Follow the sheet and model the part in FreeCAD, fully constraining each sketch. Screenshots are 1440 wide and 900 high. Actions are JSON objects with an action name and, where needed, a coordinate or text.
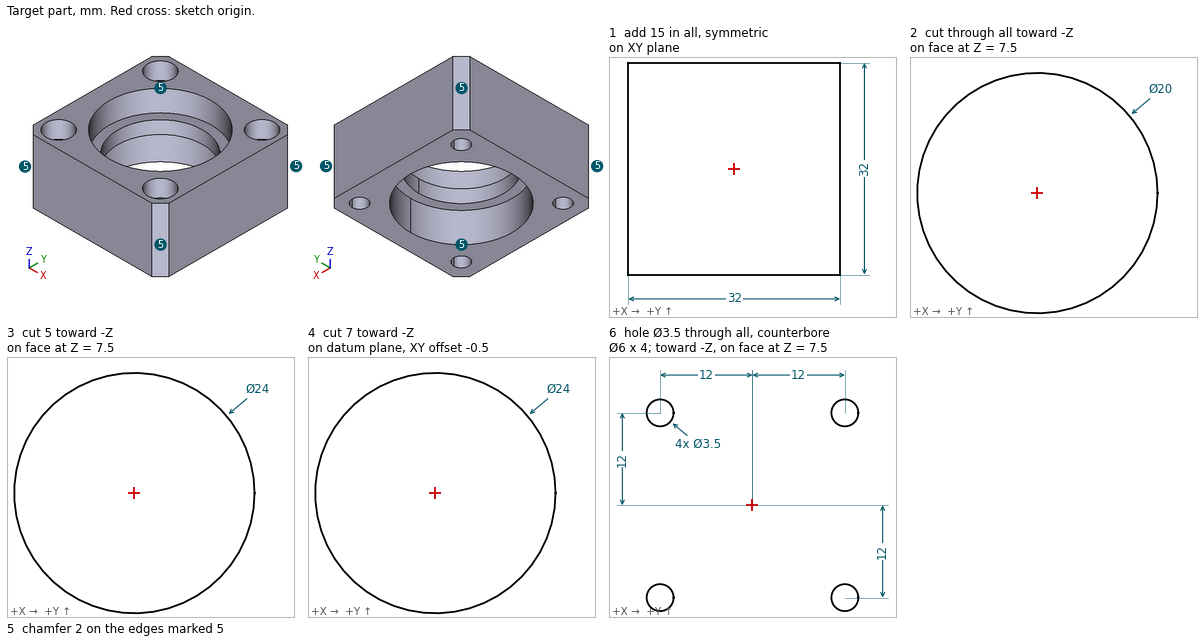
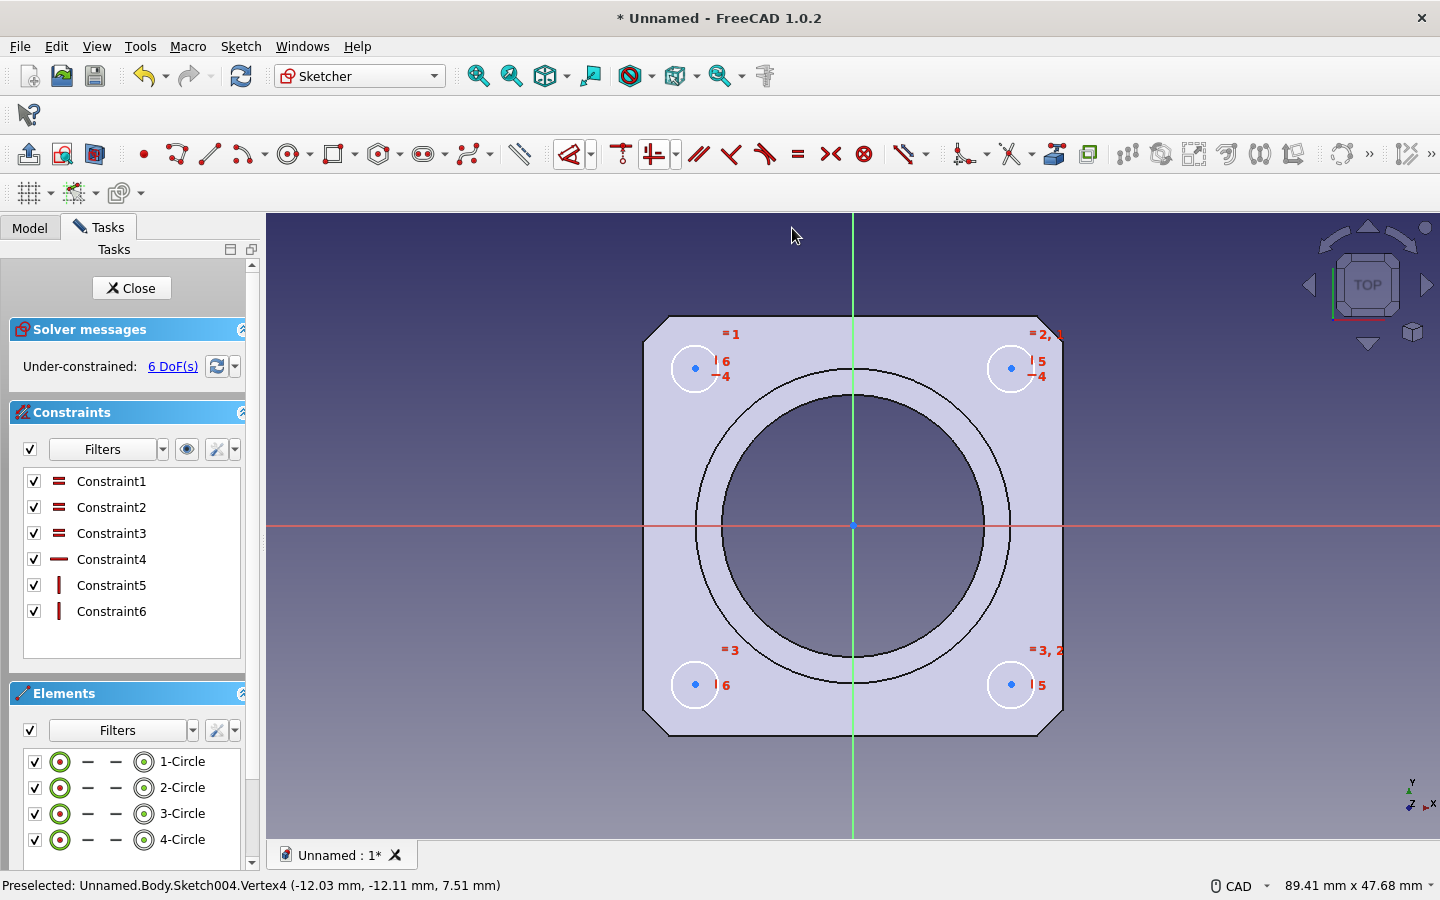
{"action": "left_click", "coordinate": [1011, 685]}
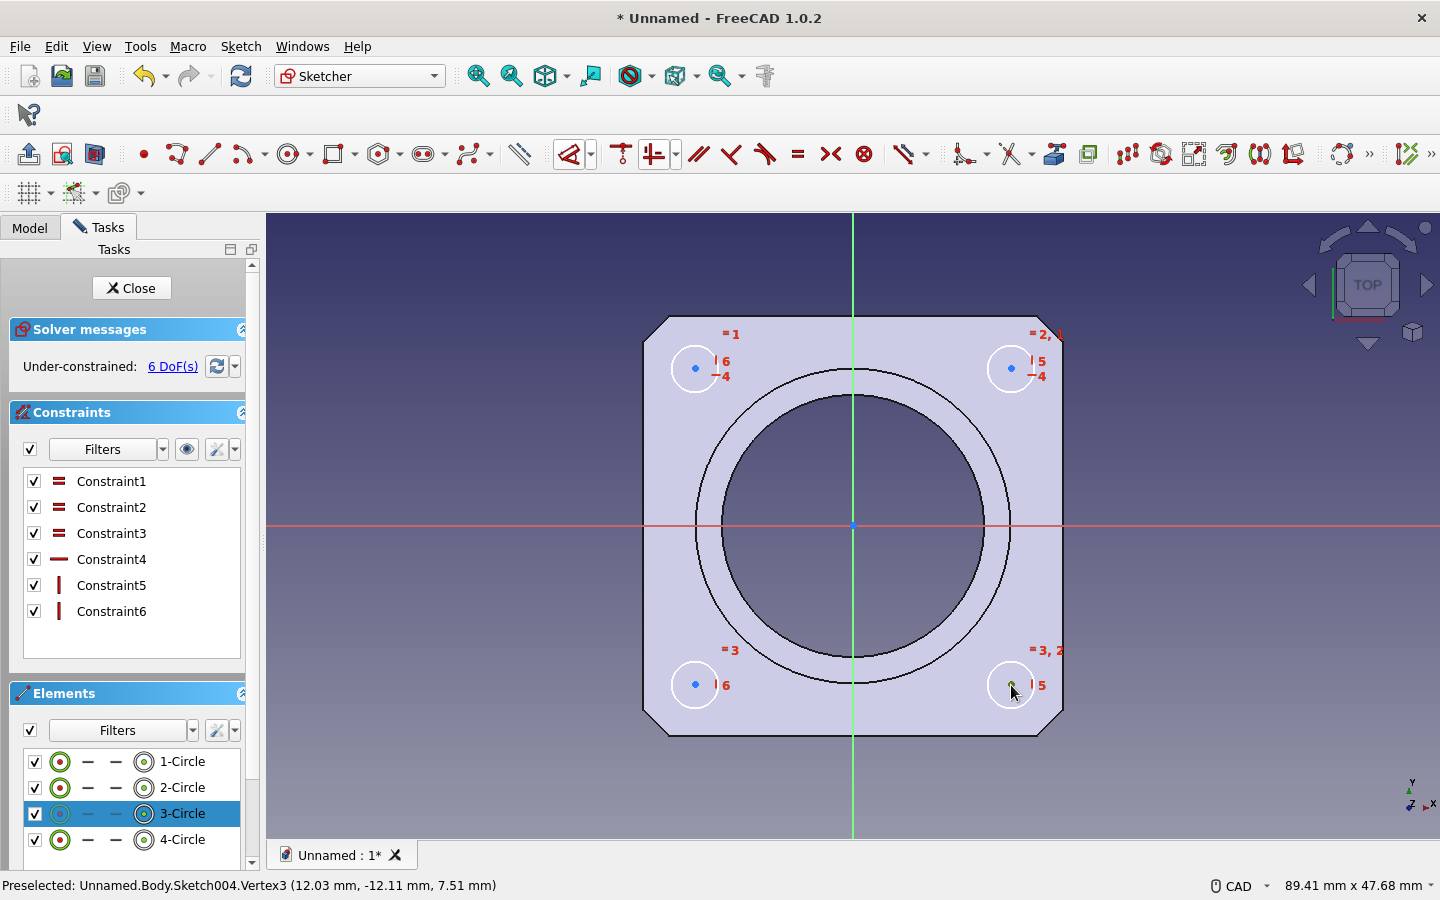
{"action": "left_click", "coordinate": [695, 685]}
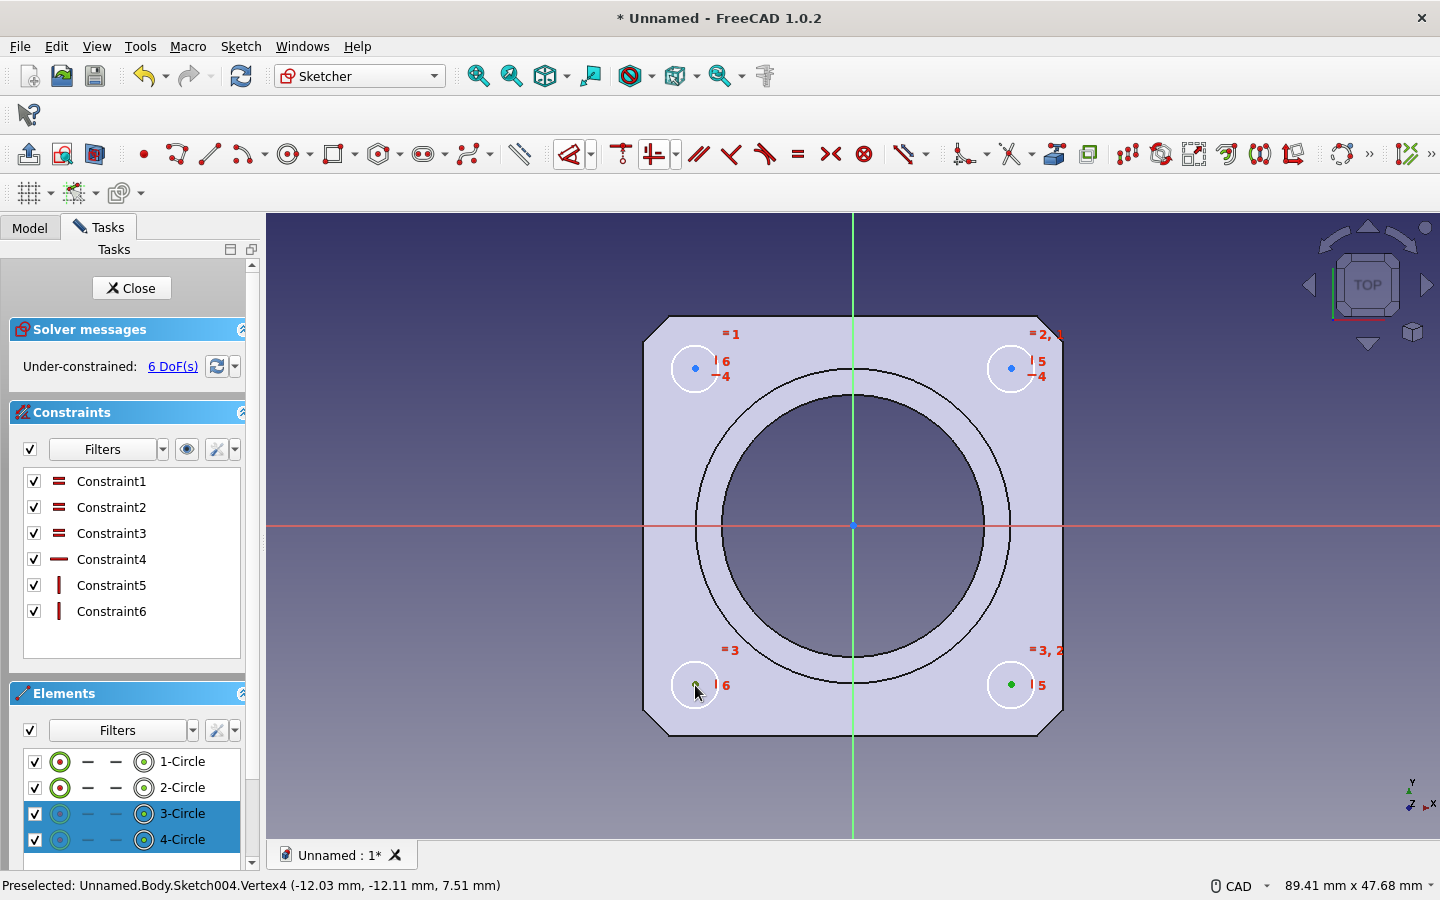
{"action": "key", "text": "h"}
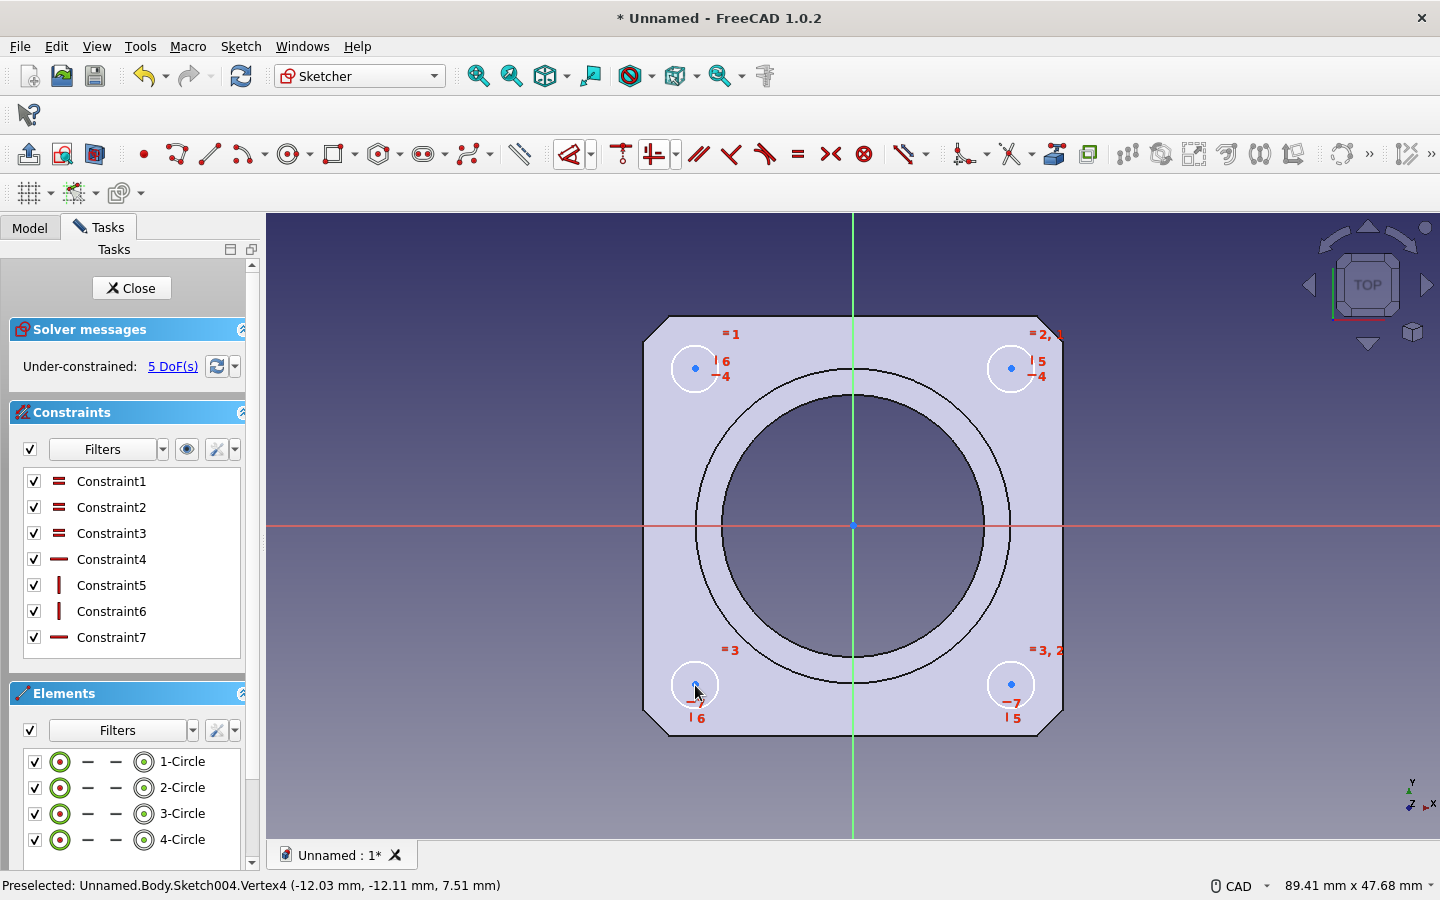
{"action": "left_click", "coordinate": [711, 352]}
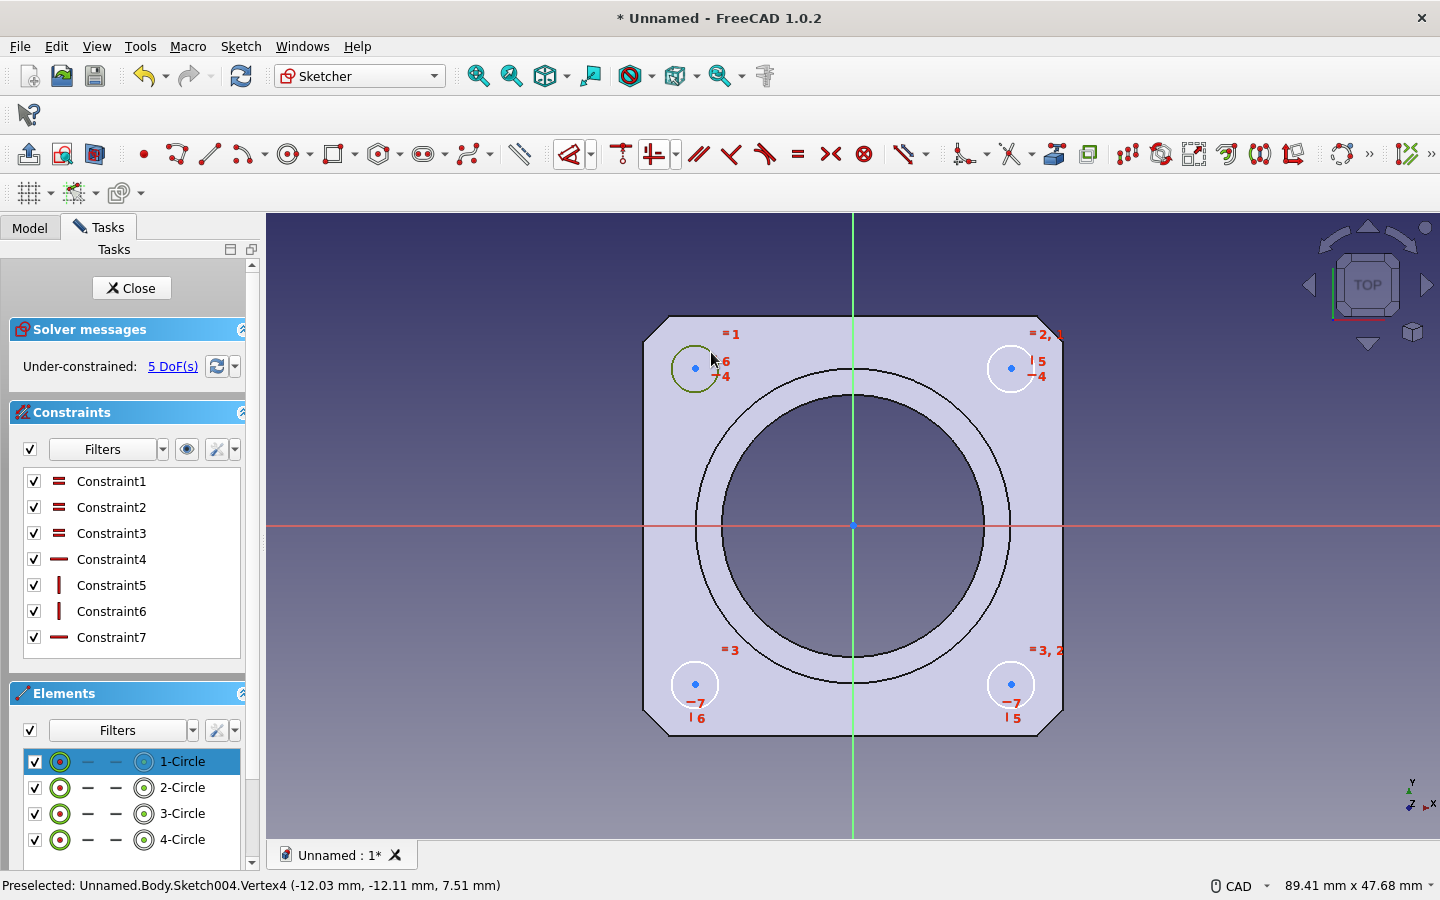
{"action": "left_click", "coordinate": [590, 154]}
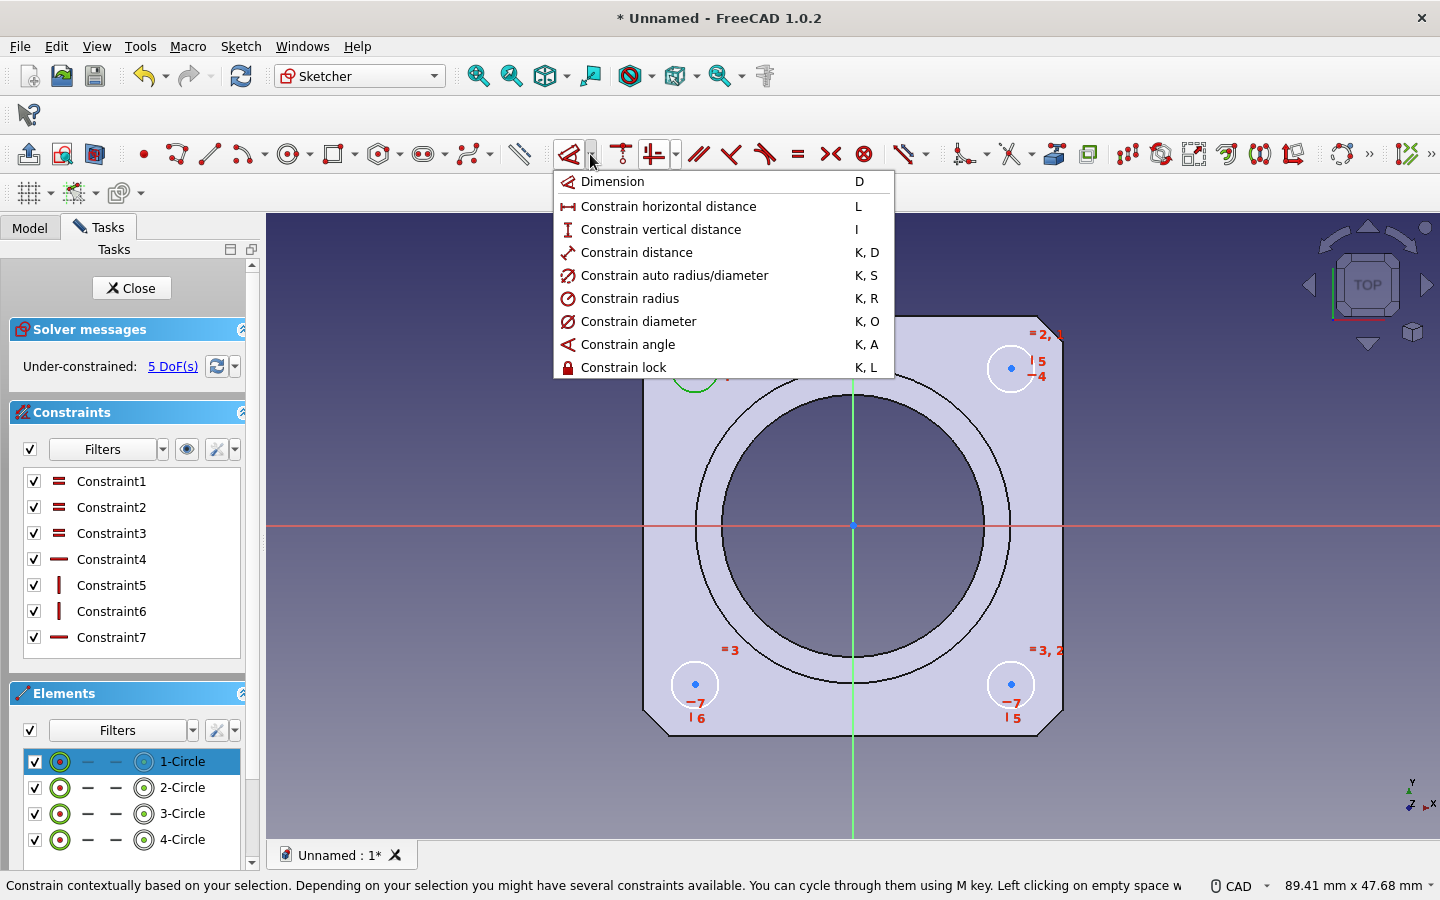
{"action": "left_click", "coordinate": [724, 322]}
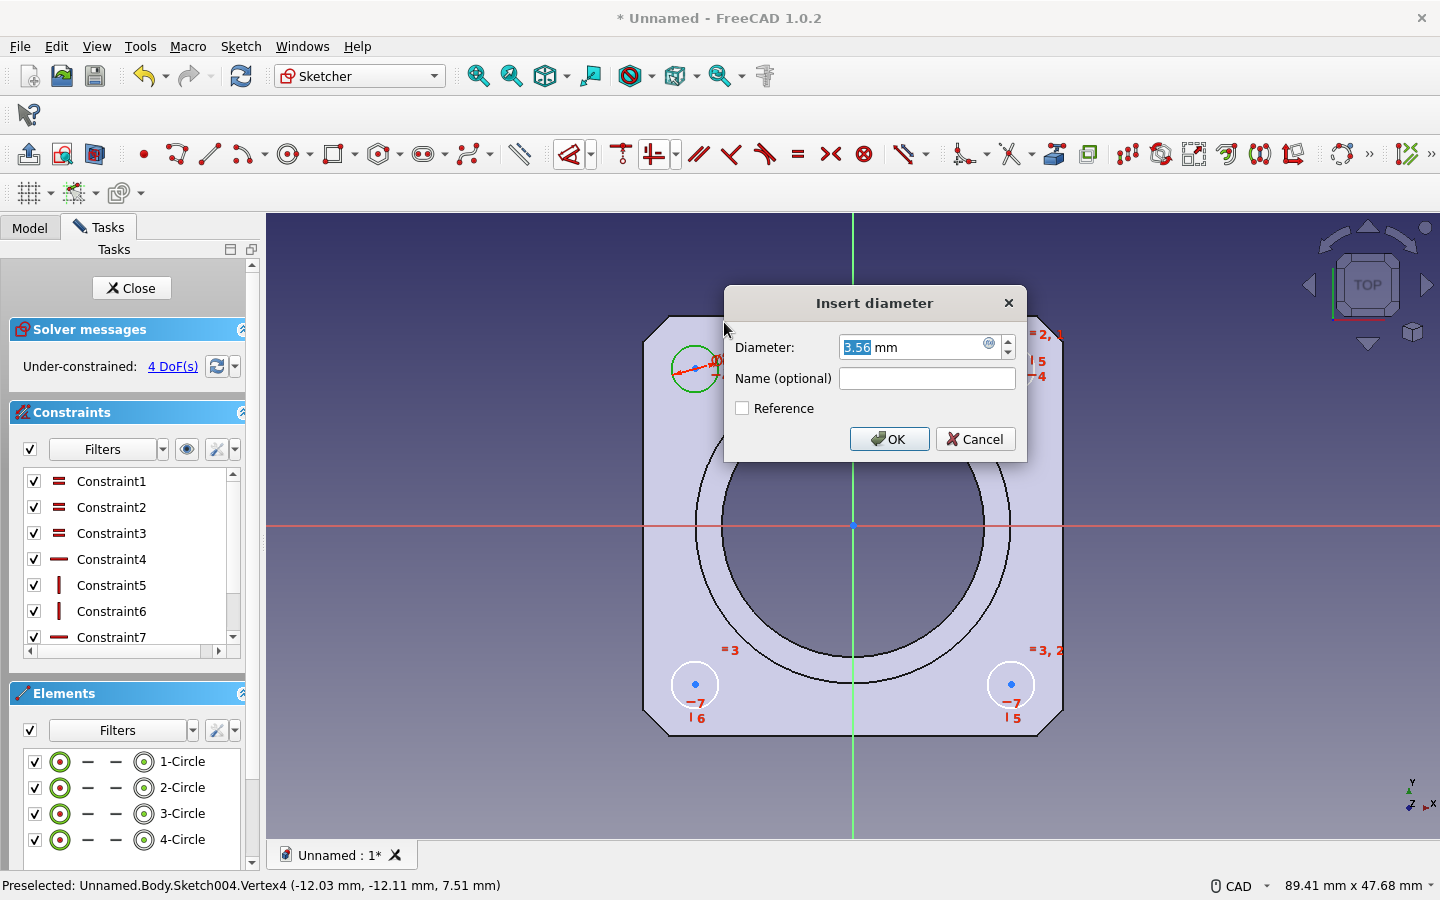
{"action": "type", "text": "3.5"}
{"action": "key", "text": "Return"}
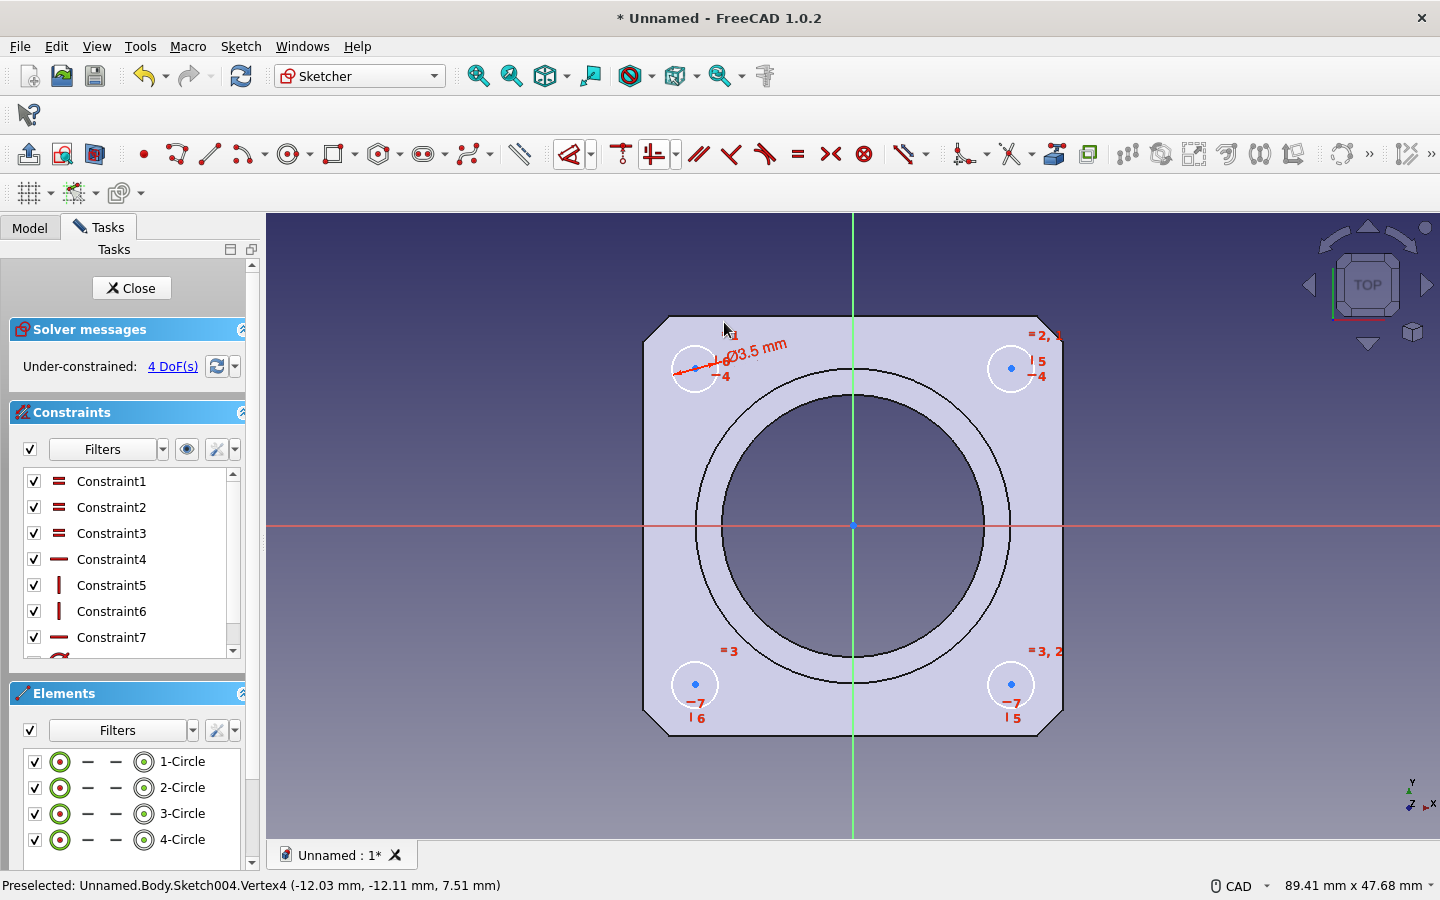
{"action": "left_click", "coordinate": [695, 369]}